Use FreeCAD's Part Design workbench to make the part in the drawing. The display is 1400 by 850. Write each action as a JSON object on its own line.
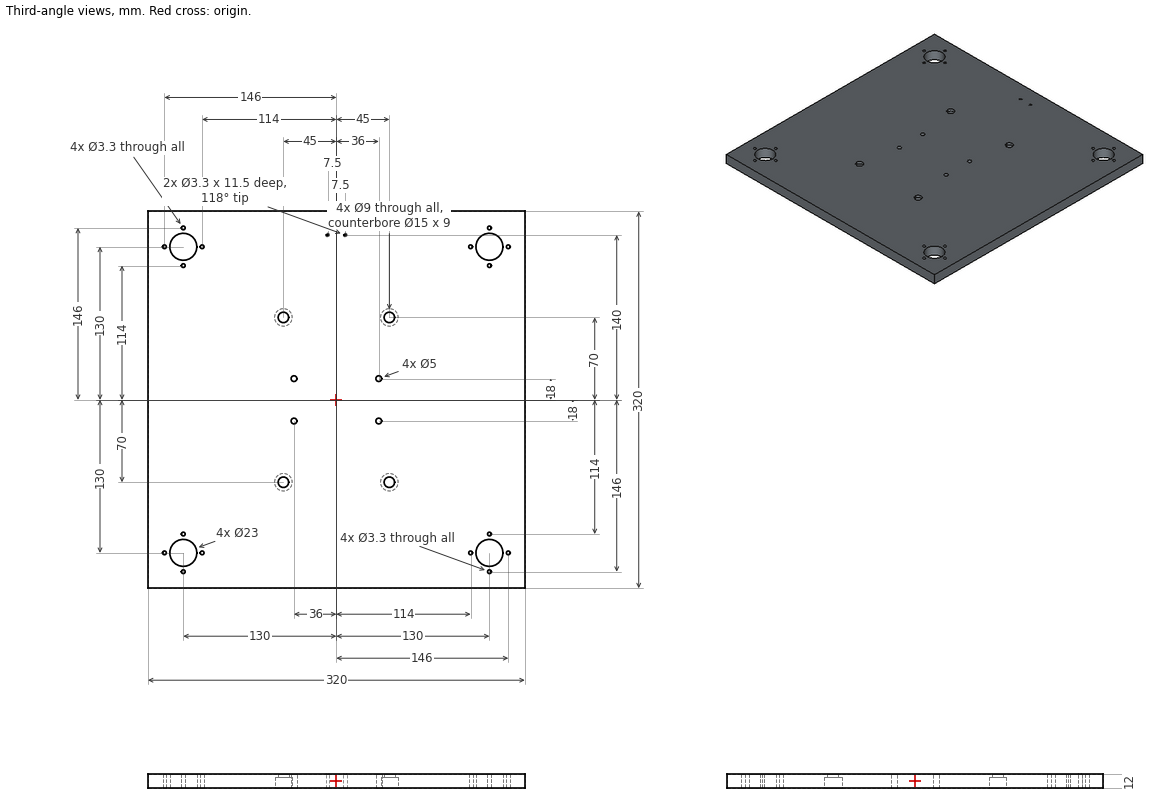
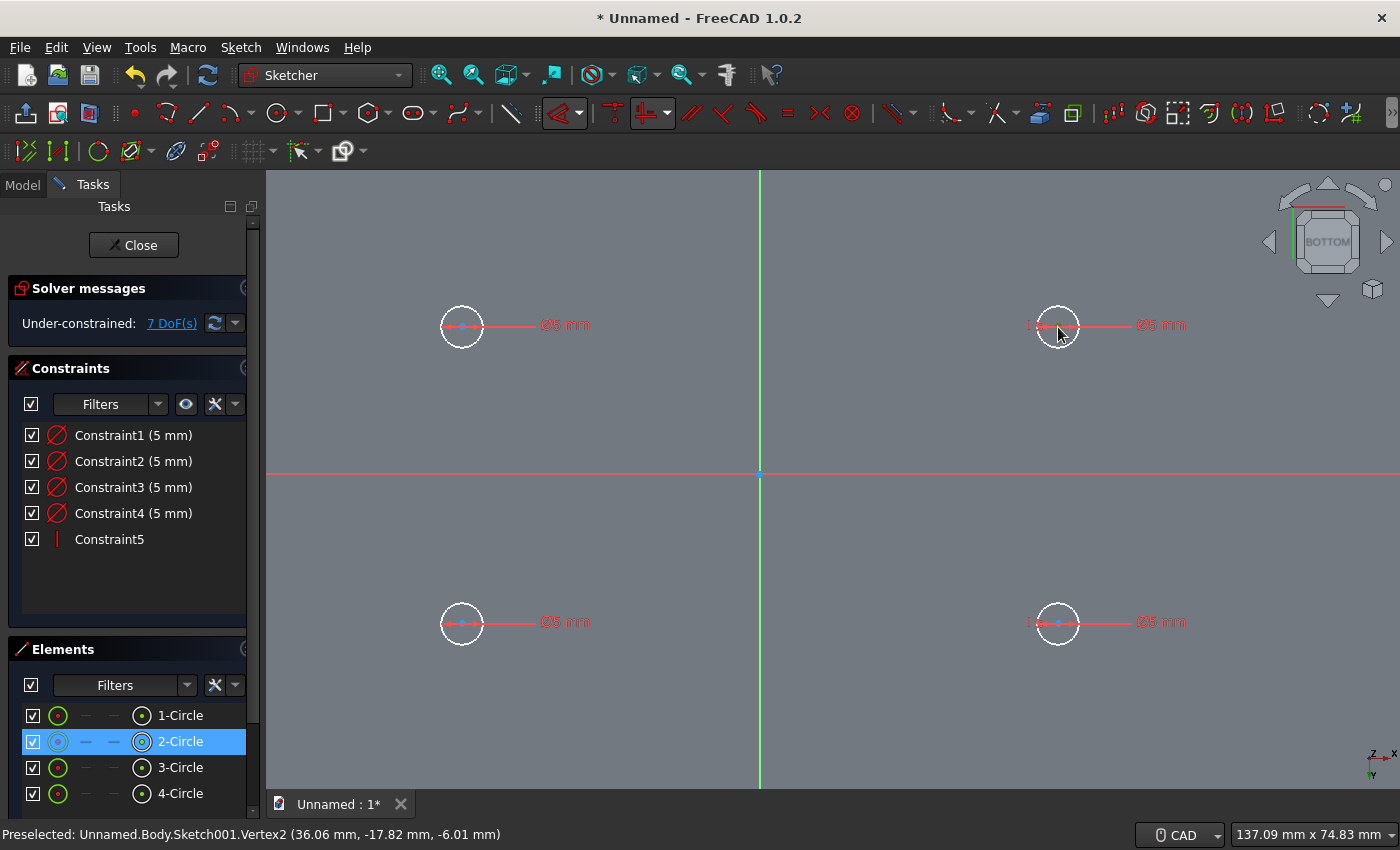
{"action": "left_click", "coordinate": [462, 327]}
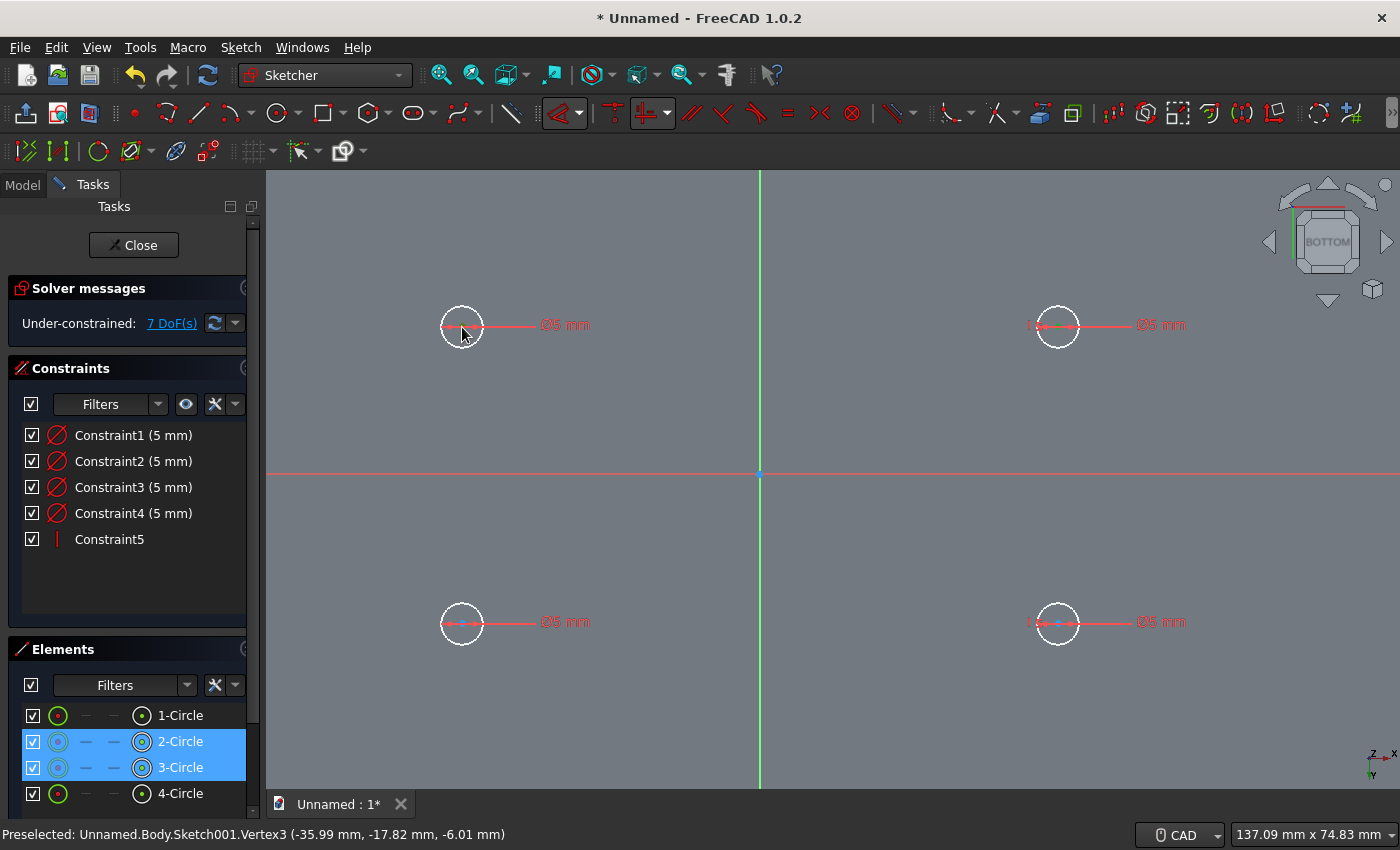
{"action": "left_click", "coordinate": [670, 114]}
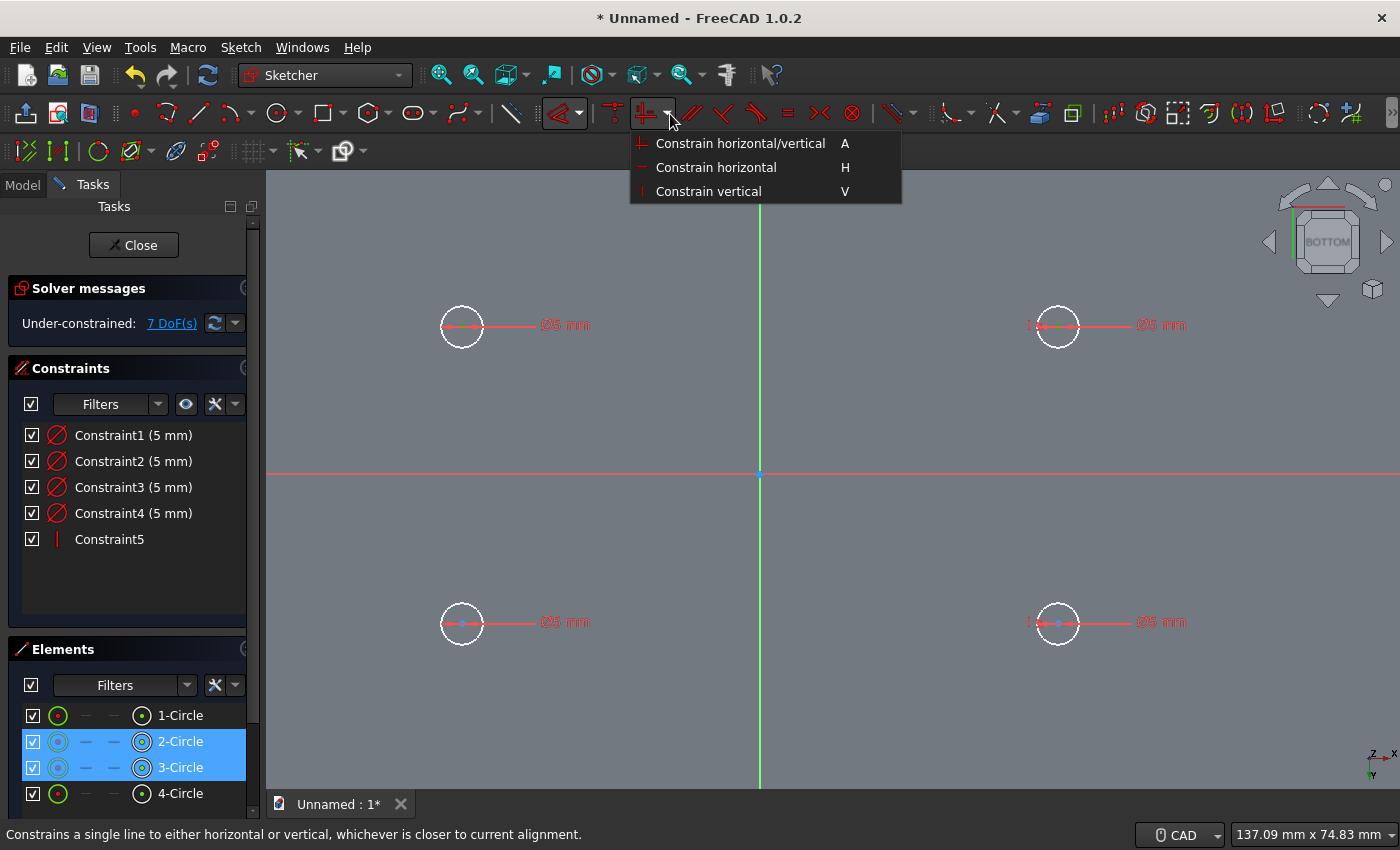
{"action": "left_click", "coordinate": [766, 167]}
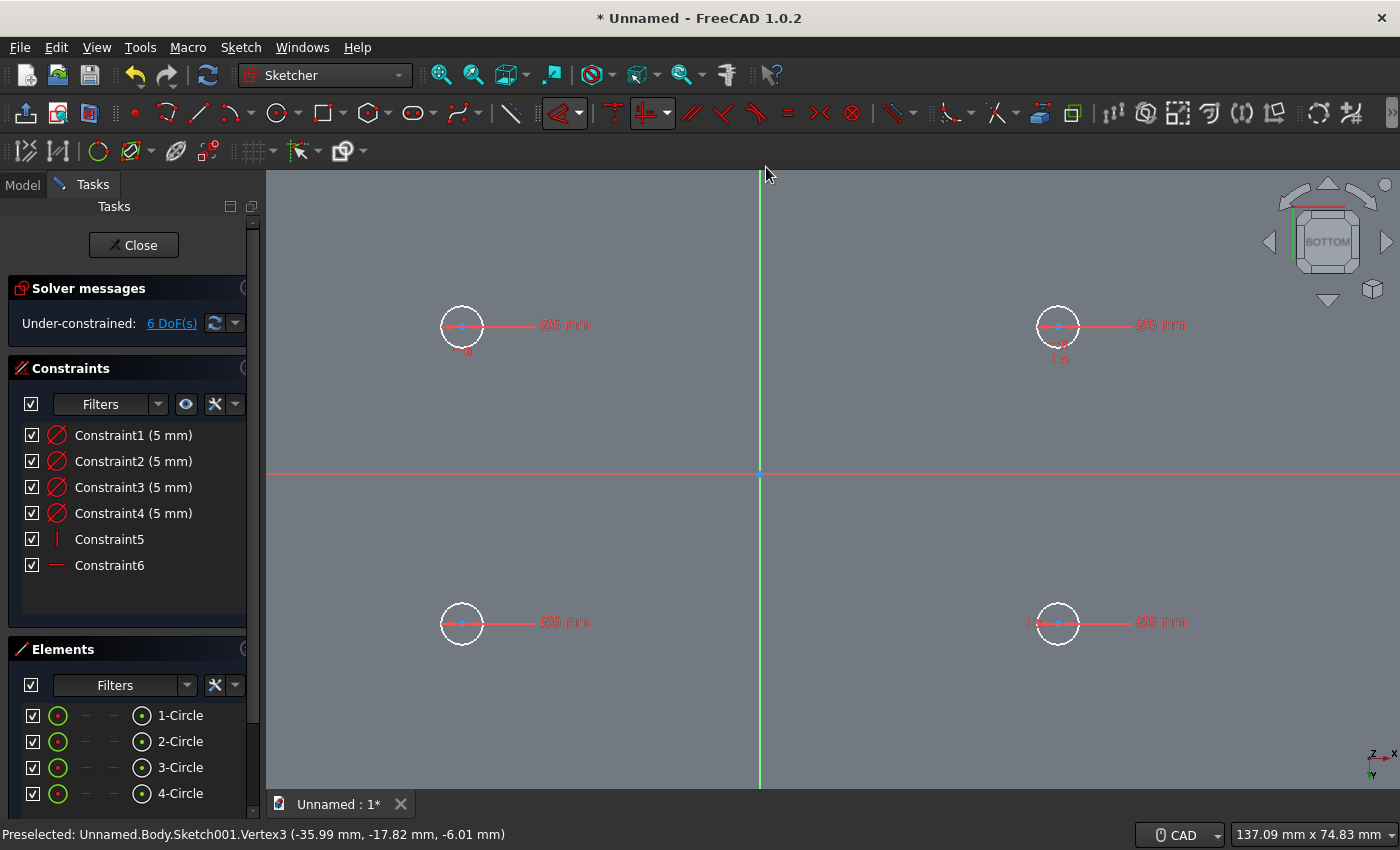
{"action": "left_click", "coordinate": [462, 327]}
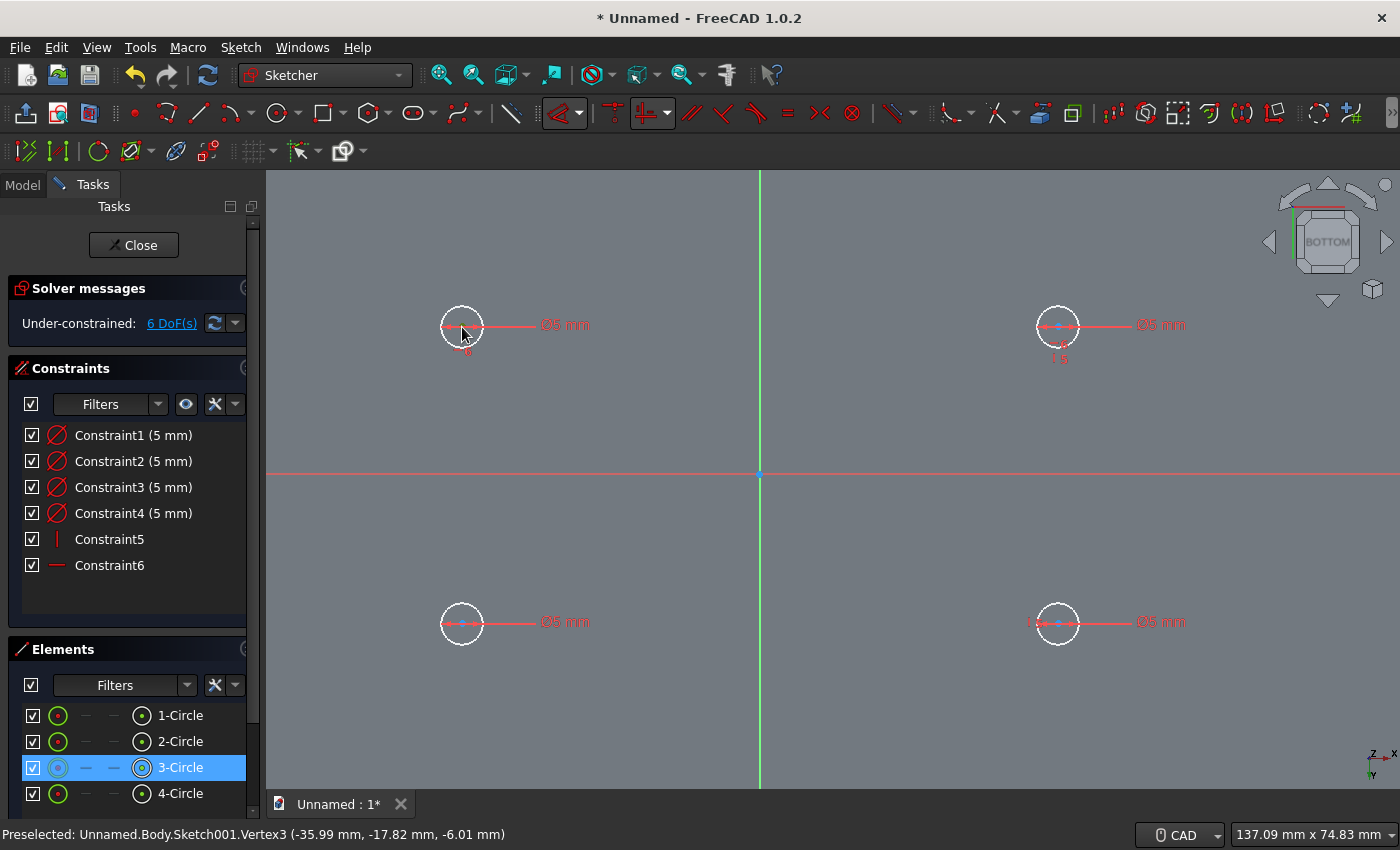
{"action": "left_click", "coordinate": [462, 624]}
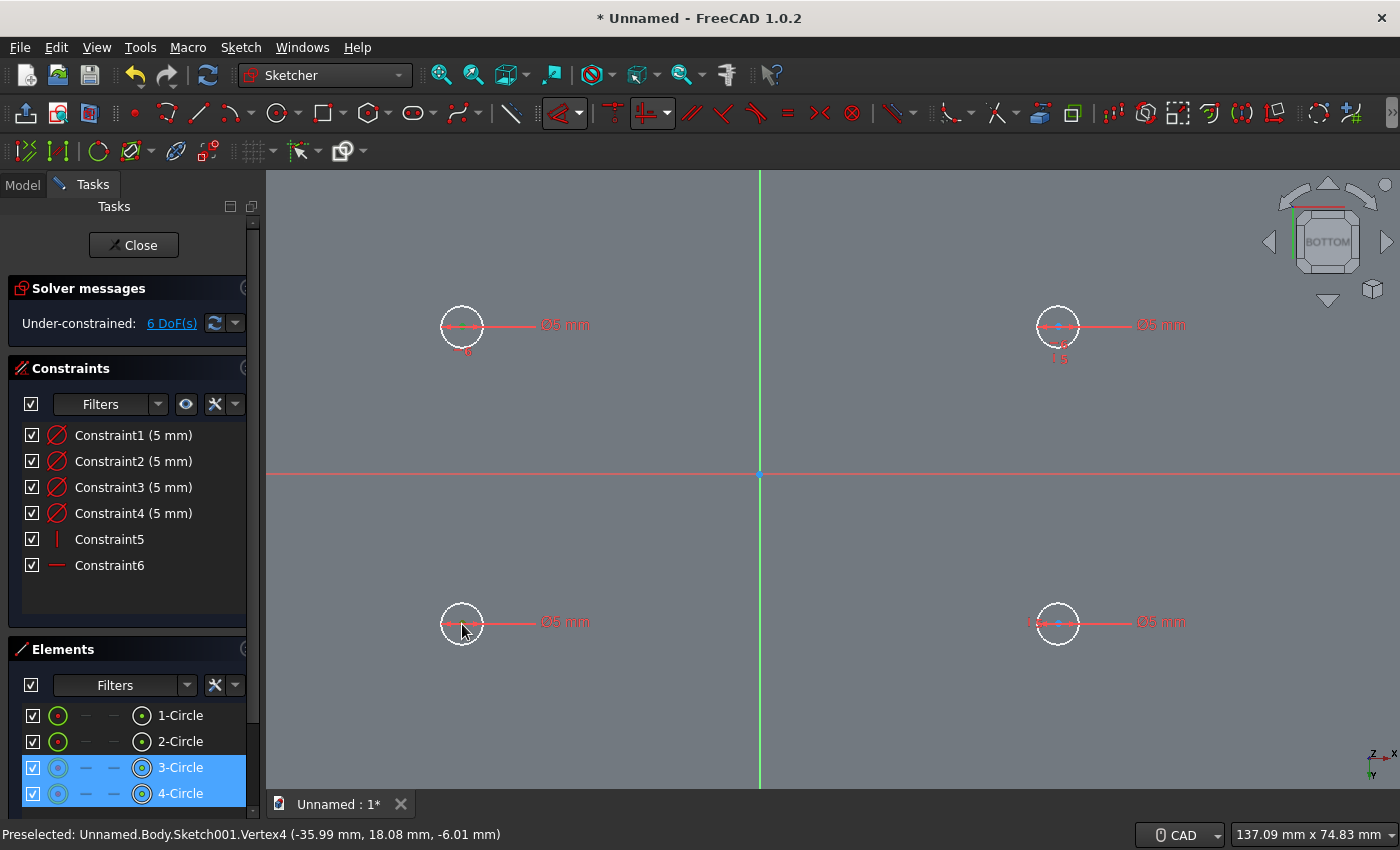
{"action": "left_click", "coordinate": [670, 114]}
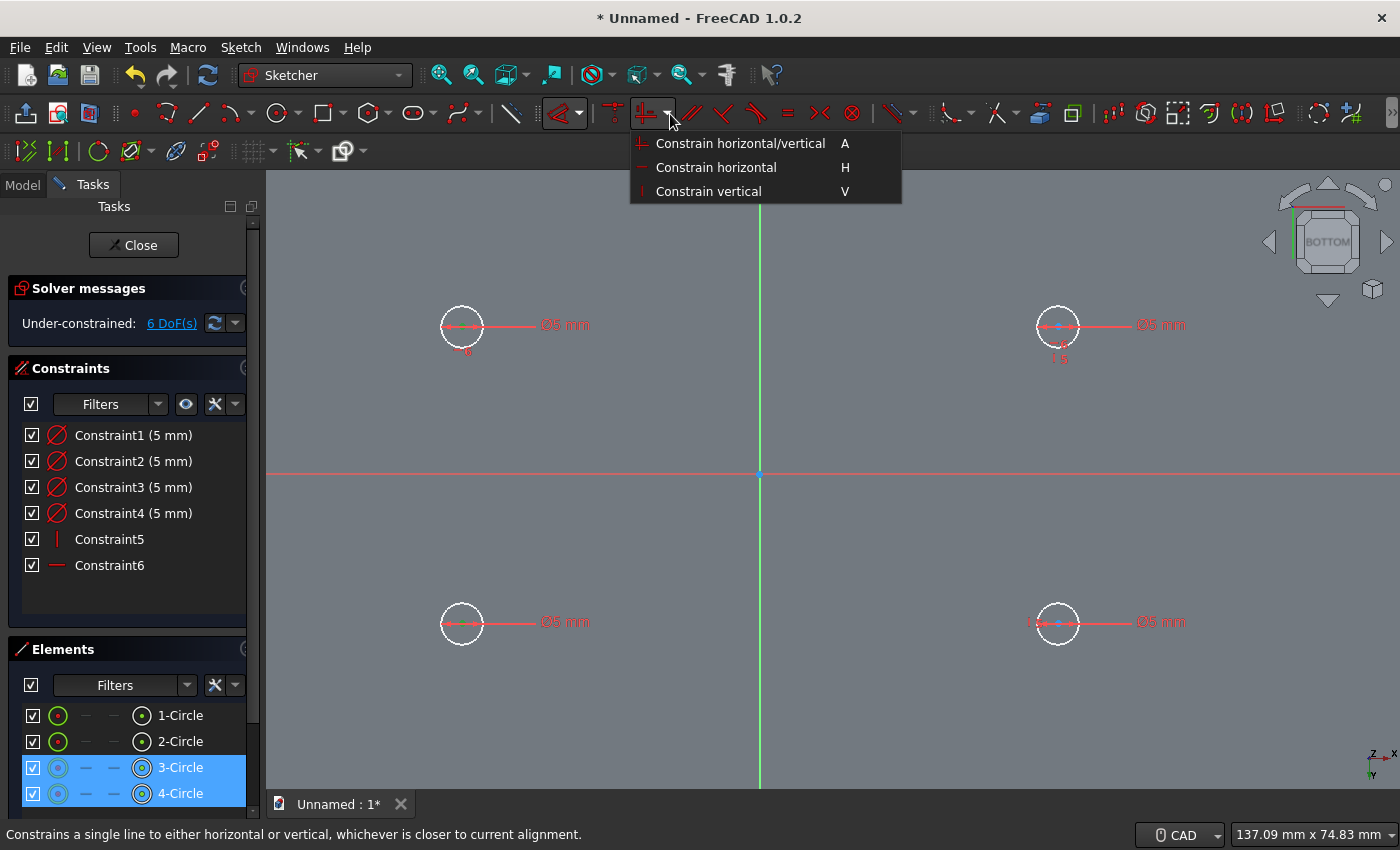
{"action": "left_click", "coordinate": [766, 191]}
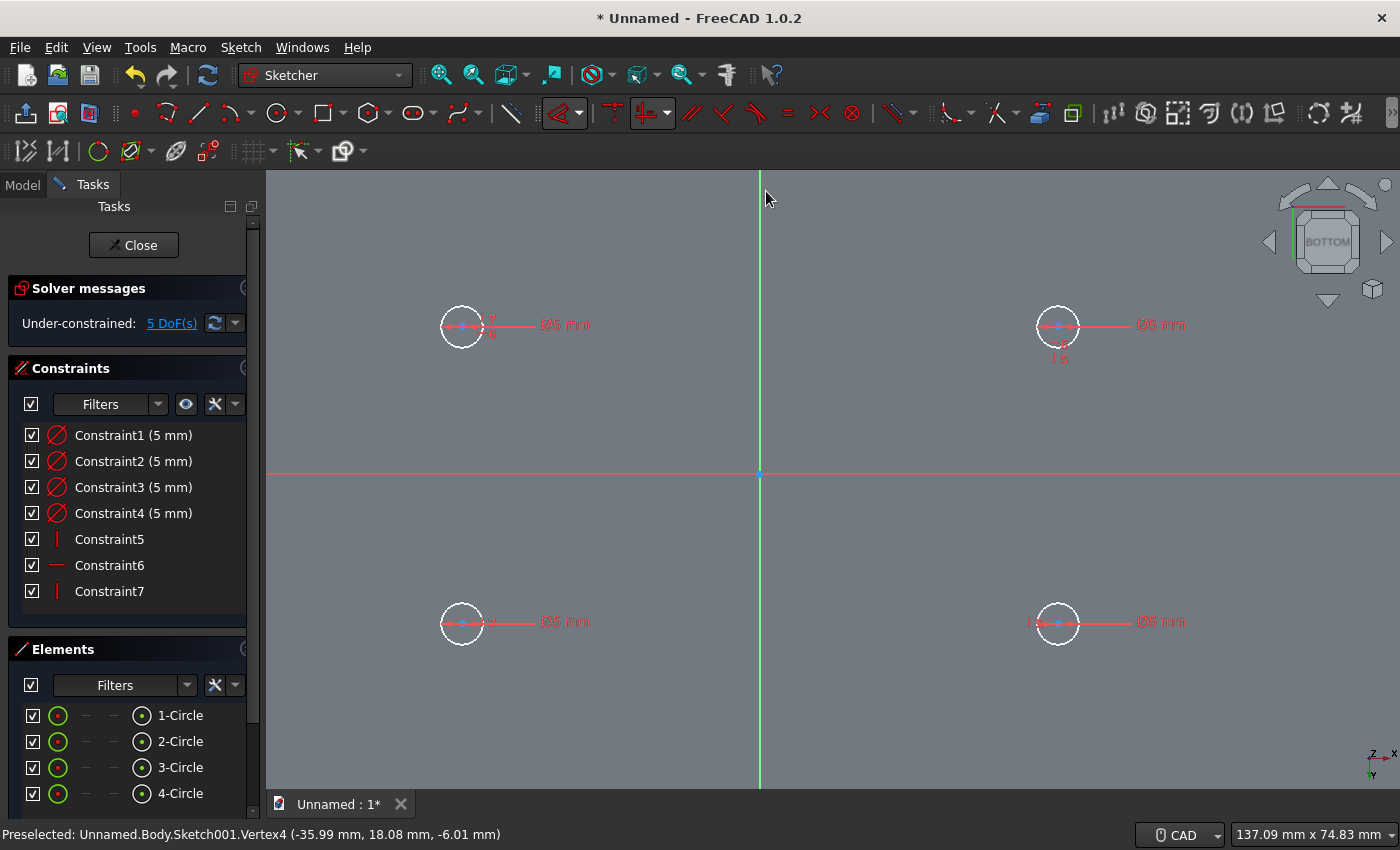
{"action": "left_click", "coordinate": [1058, 624]}